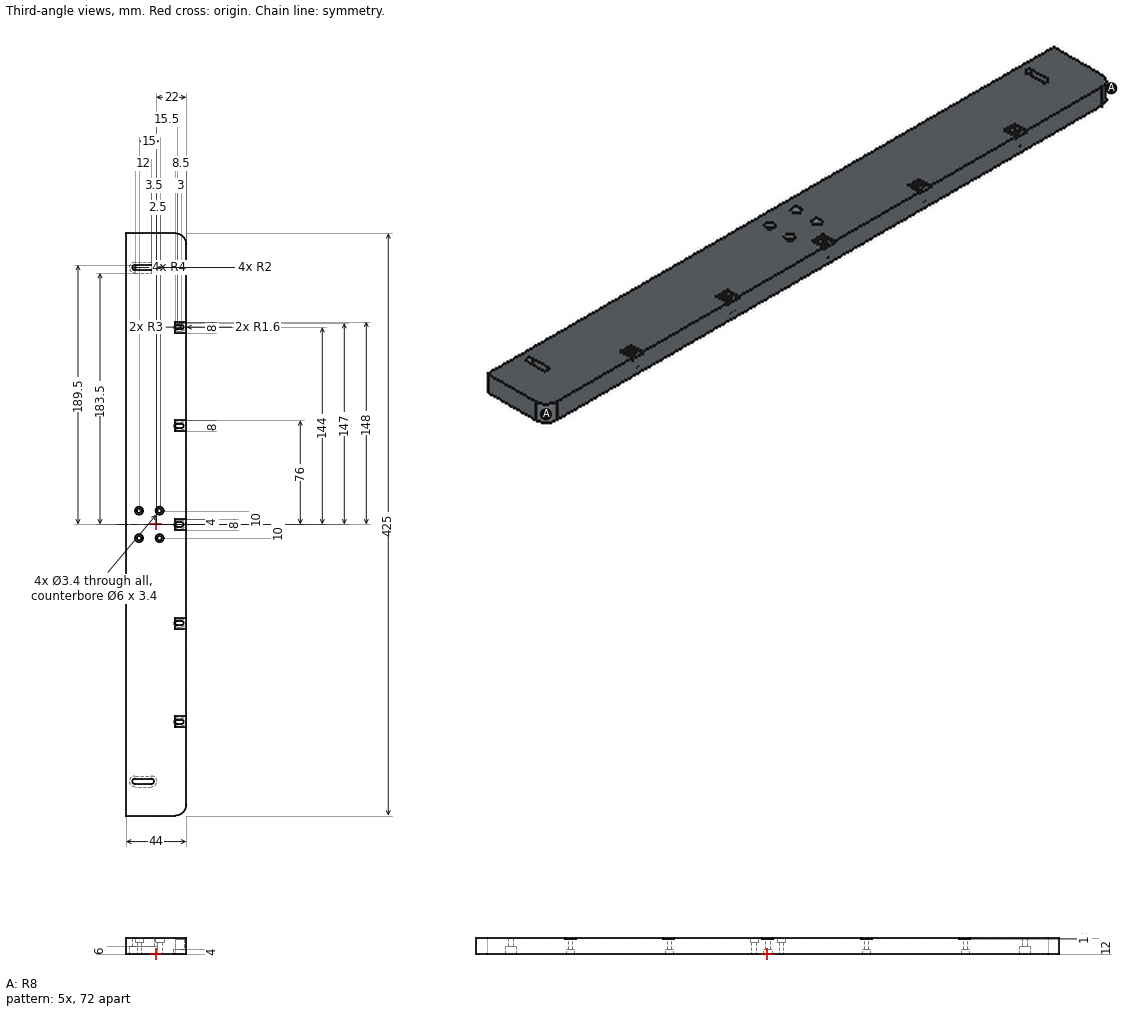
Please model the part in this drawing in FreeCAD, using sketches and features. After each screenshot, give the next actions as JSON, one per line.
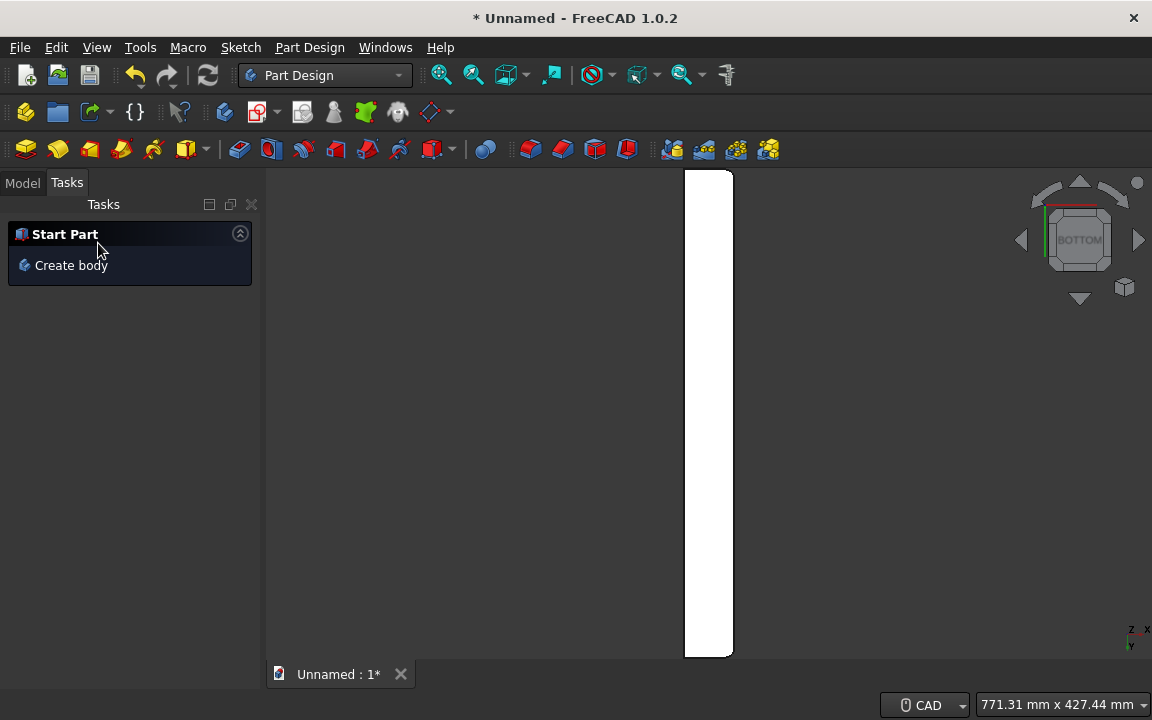
{"action": "left_click", "coordinate": [709, 622]}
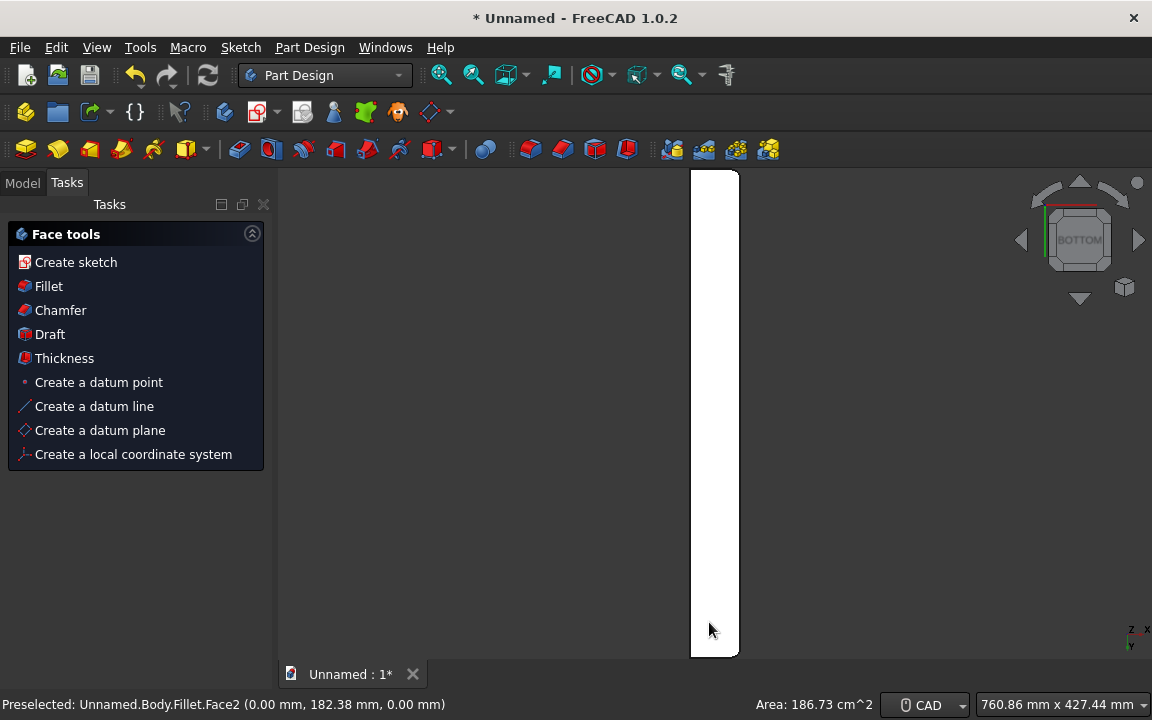
{"action": "left_click", "coordinate": [258, 112]}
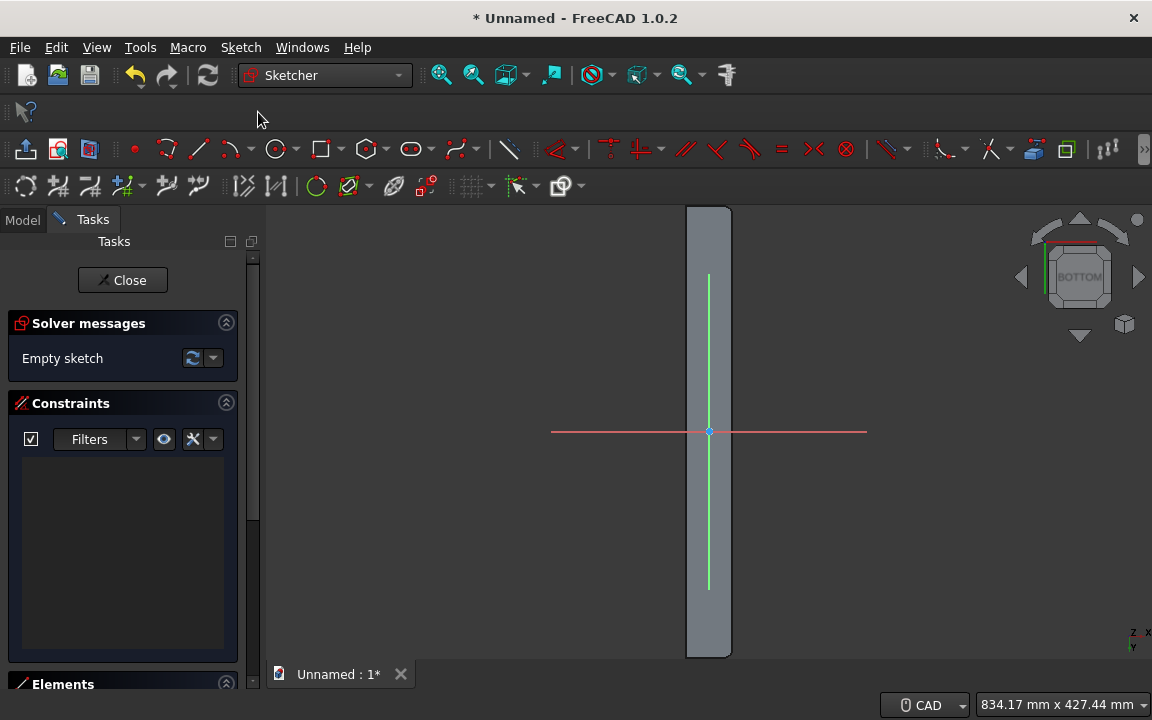
{"action": "scroll", "coordinate": [522, 432], "scroll_direction": "down", "scroll_amount": 2}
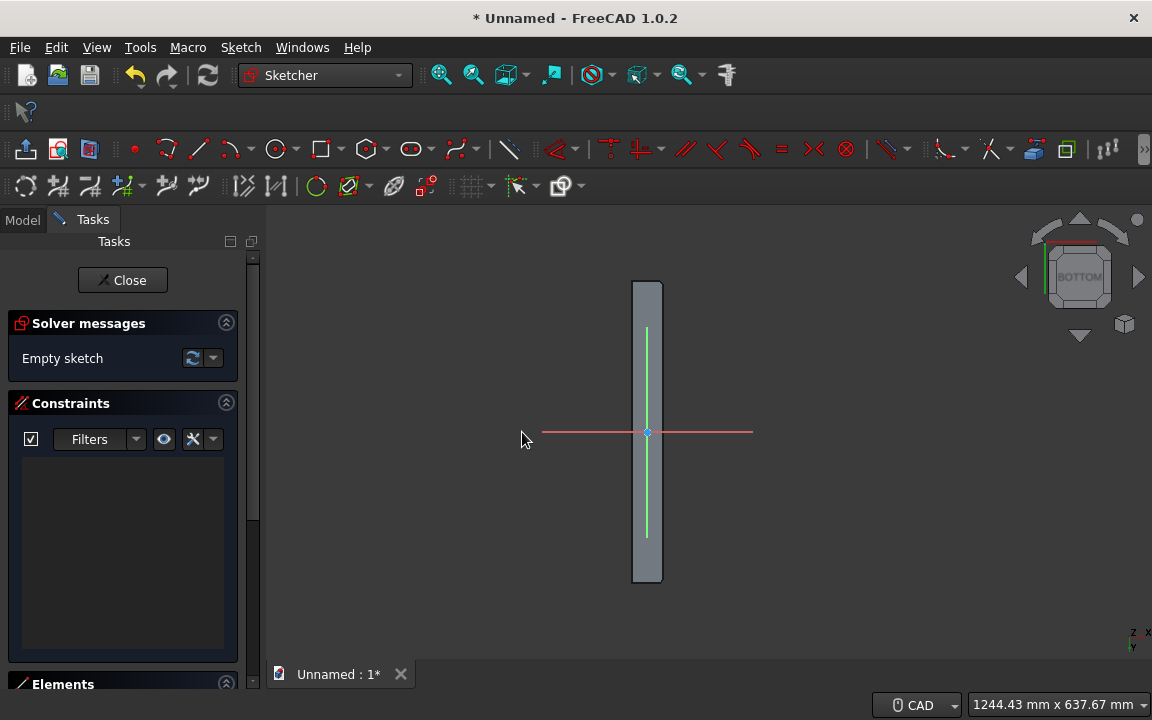
{"action": "key", "text": "g s"}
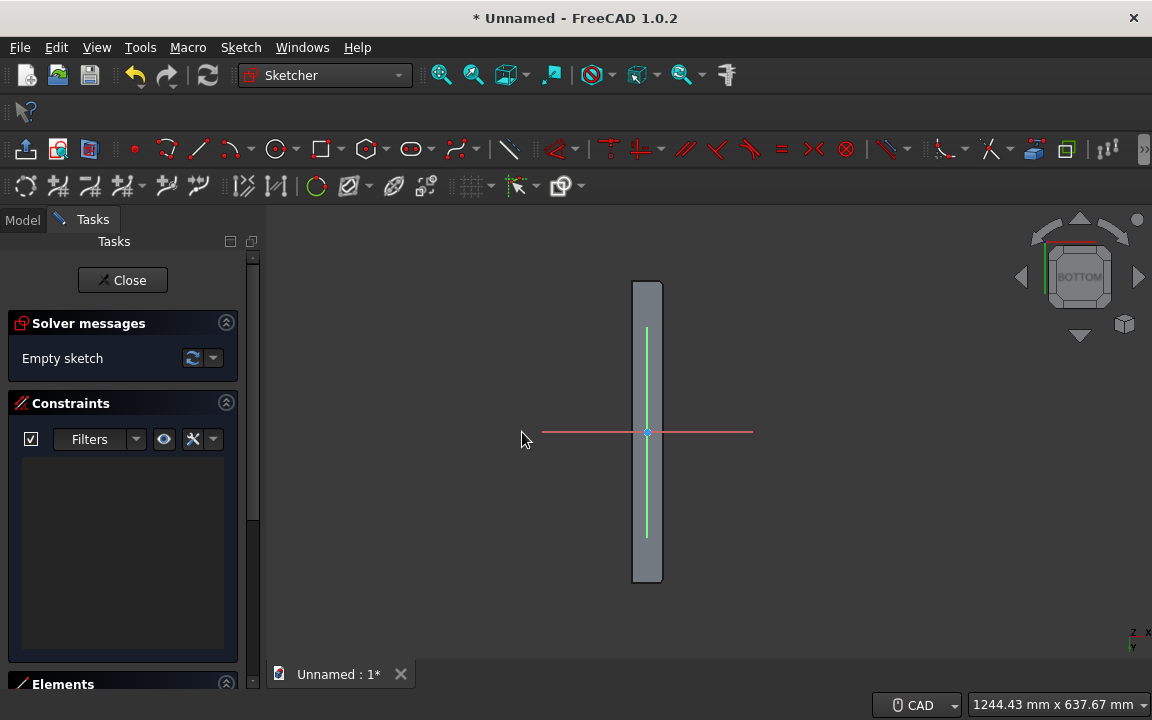
{"action": "scroll", "coordinate": [636, 566], "scroll_direction": "up", "scroll_amount": 11}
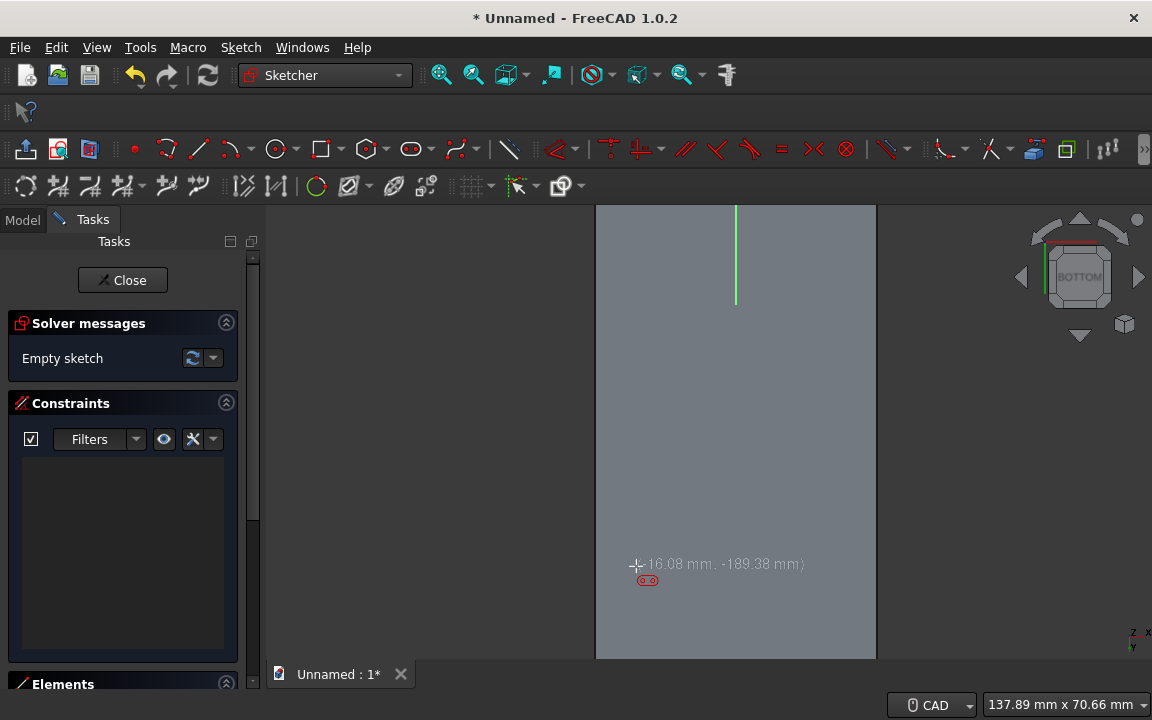
{"action": "scroll", "coordinate": [636, 567], "scroll_direction": "down", "scroll_amount": 11}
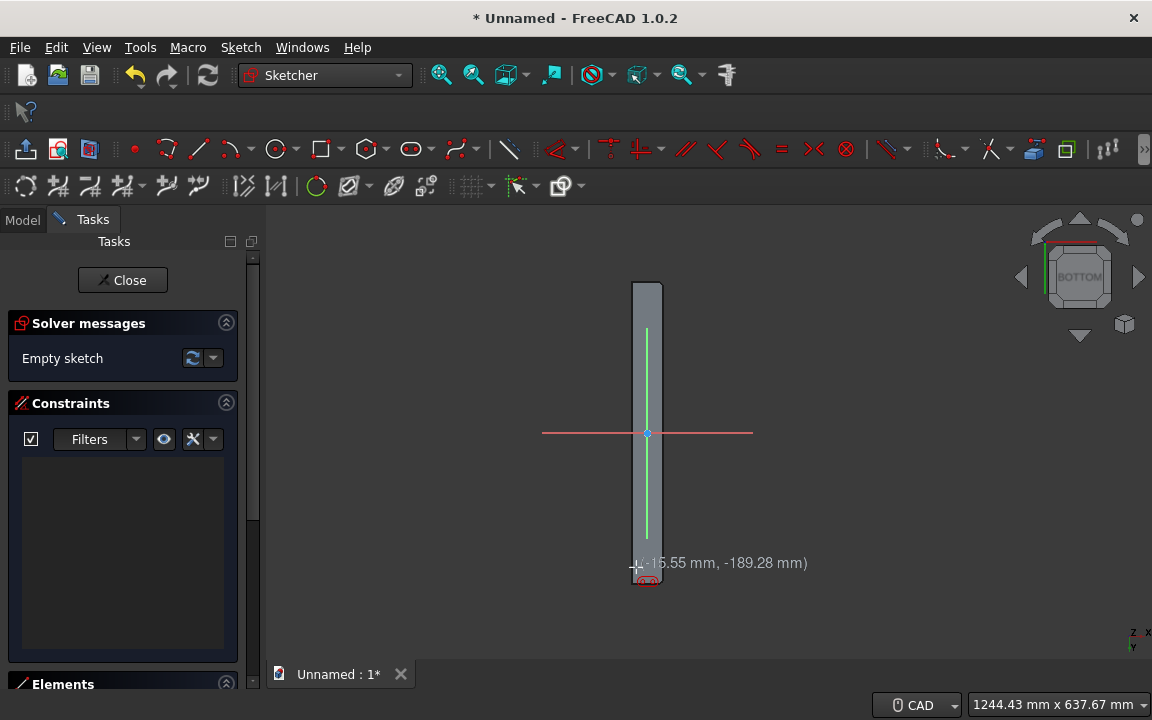
{"action": "scroll", "coordinate": [636, 567], "scroll_direction": "up", "scroll_amount": 2}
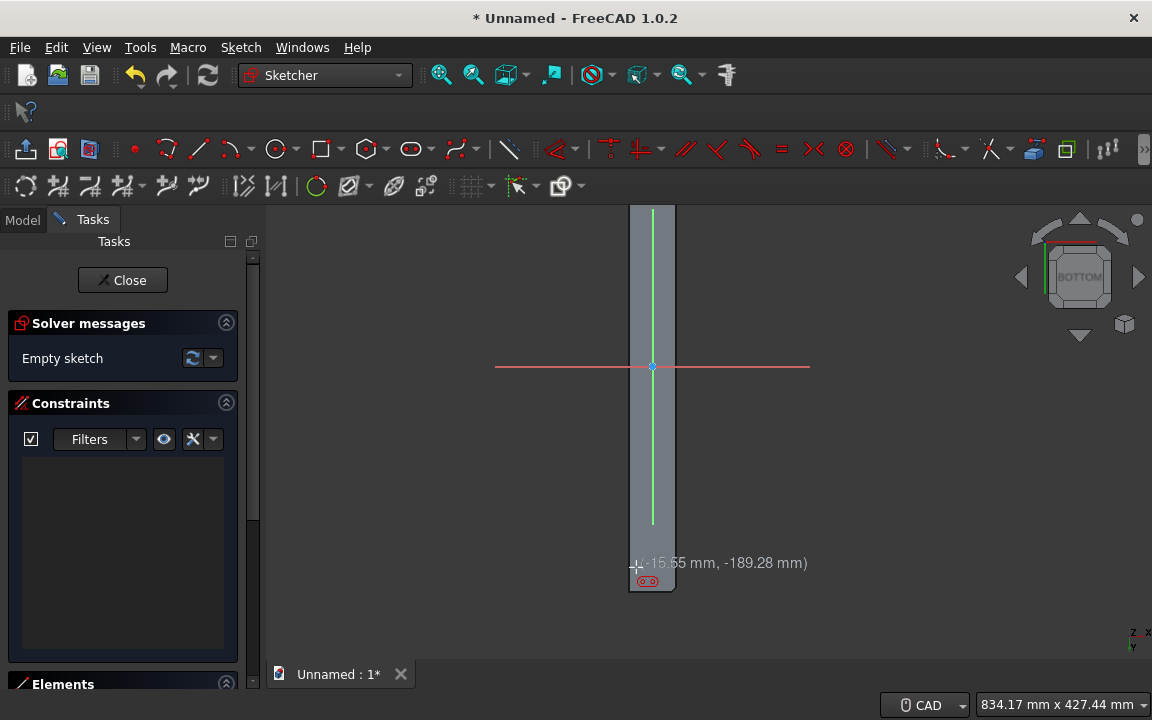
{"action": "left_click", "coordinate": [636, 566]}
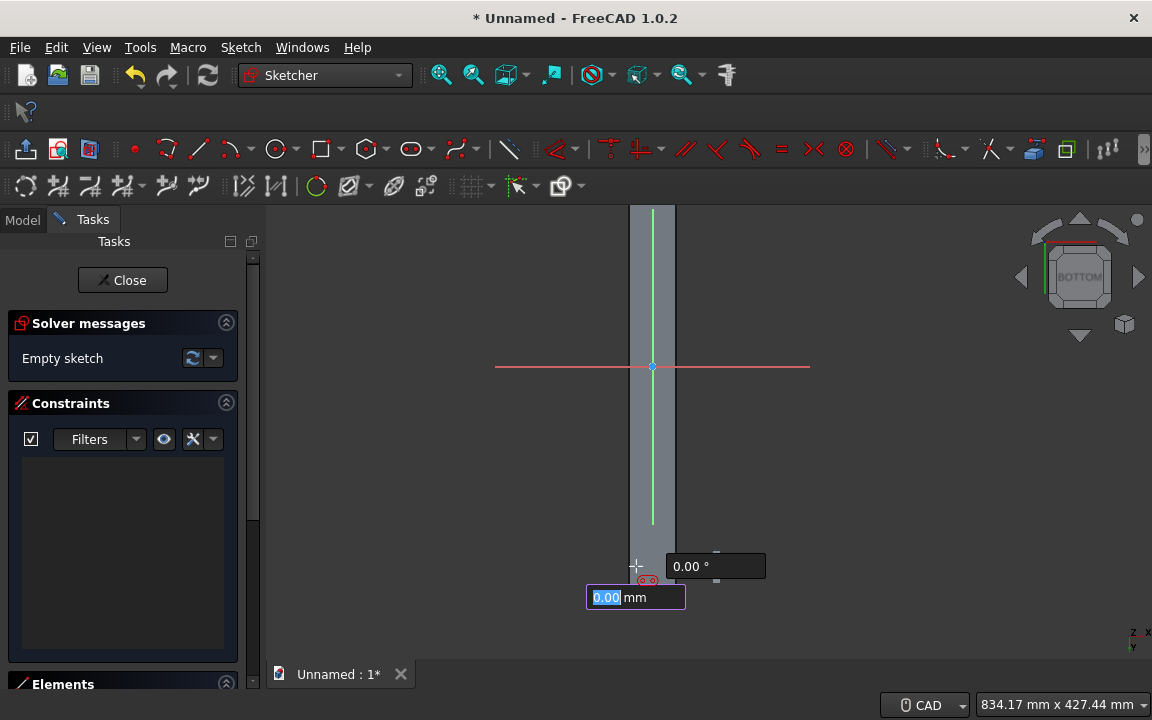
{"action": "scroll", "coordinate": [649, 566], "scroll_direction": "up", "scroll_amount": 8}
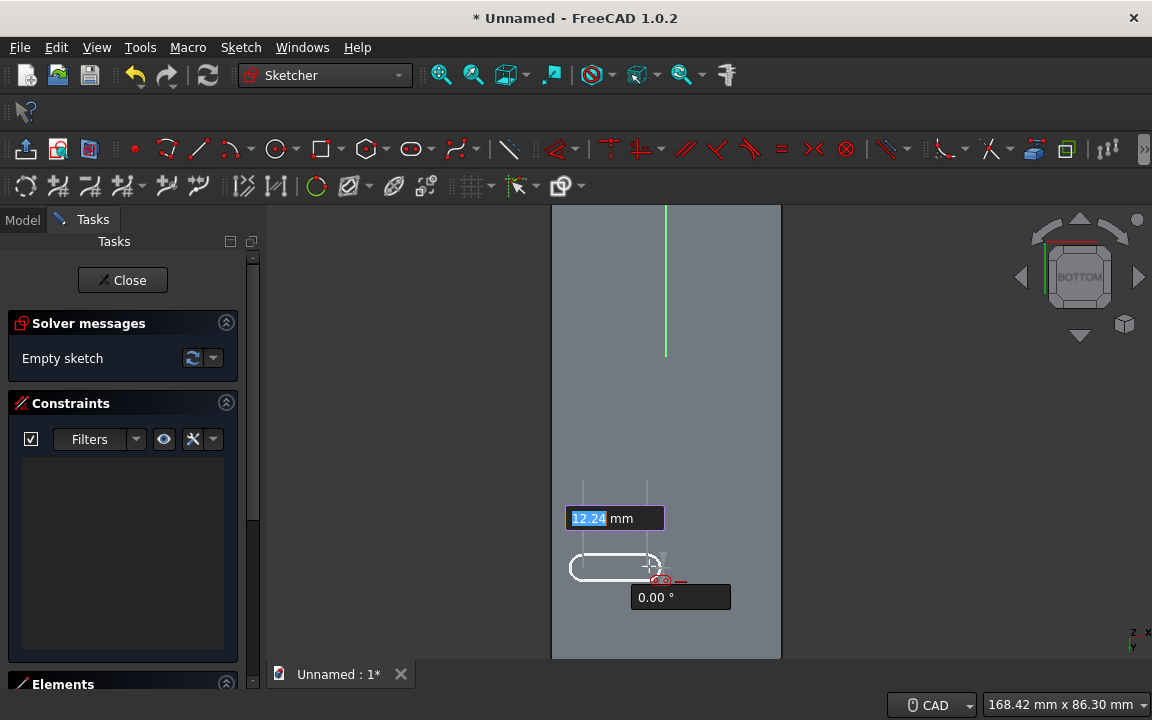
{"action": "left_click", "coordinate": [648, 563]}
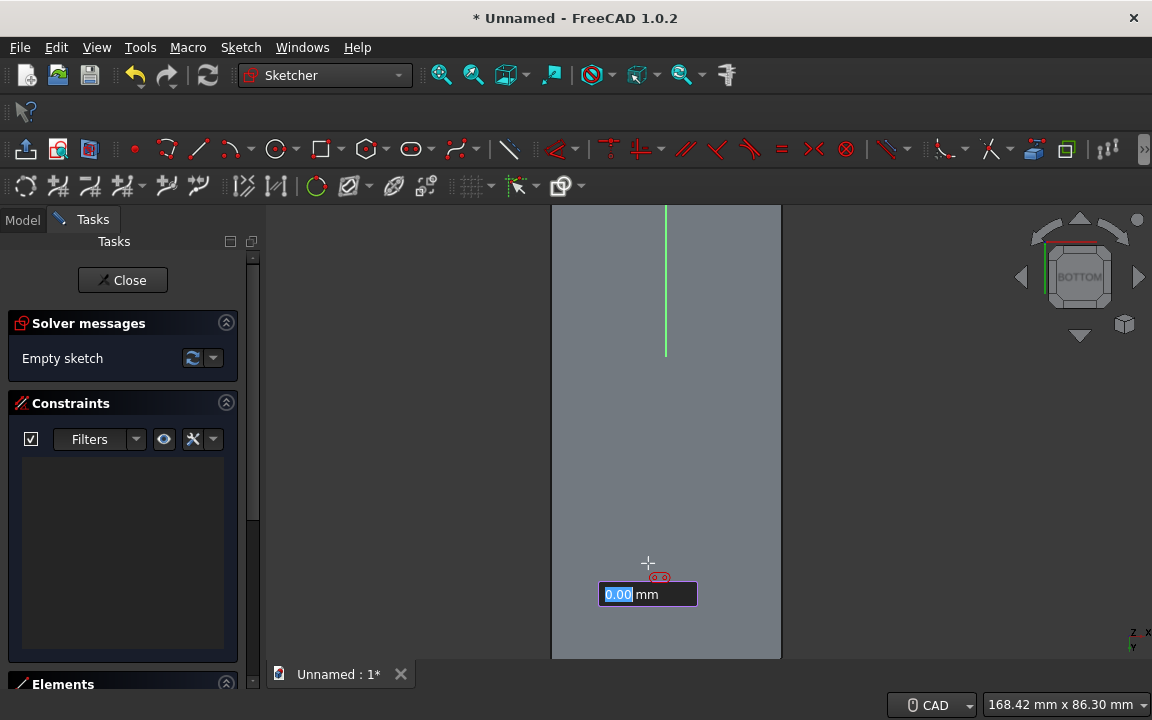
{"action": "left_click", "coordinate": [616, 541]}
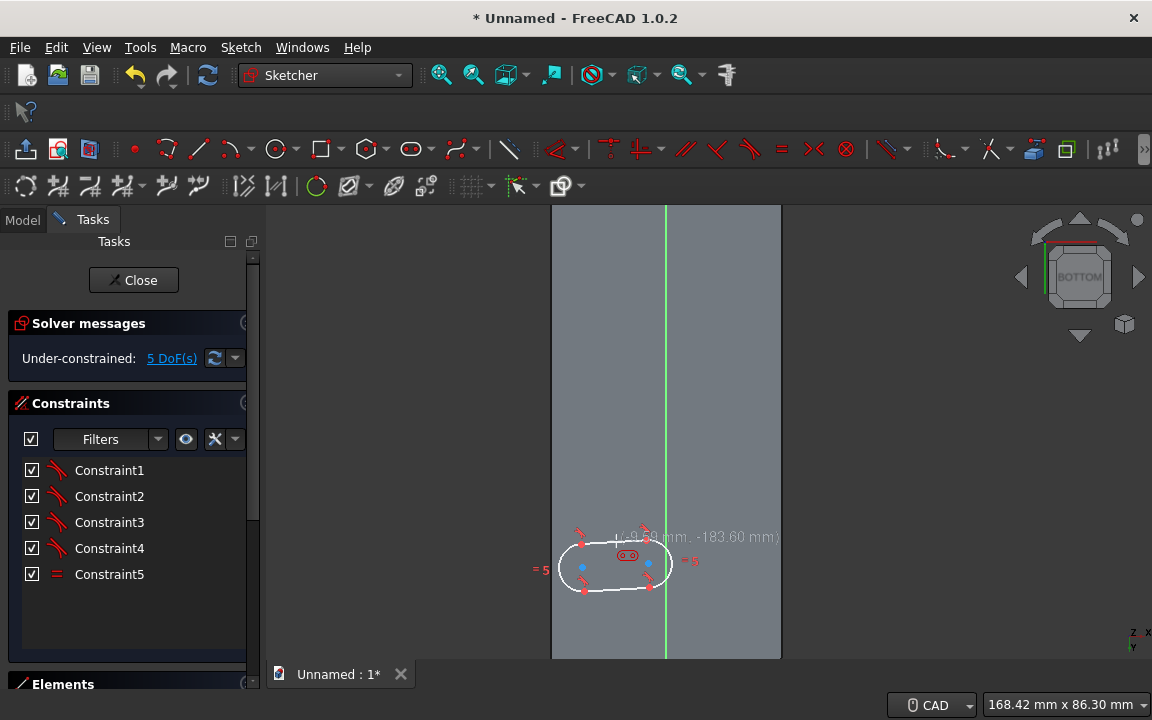
{"action": "scroll", "coordinate": [644, 566], "scroll_direction": "down", "scroll_amount": 10}